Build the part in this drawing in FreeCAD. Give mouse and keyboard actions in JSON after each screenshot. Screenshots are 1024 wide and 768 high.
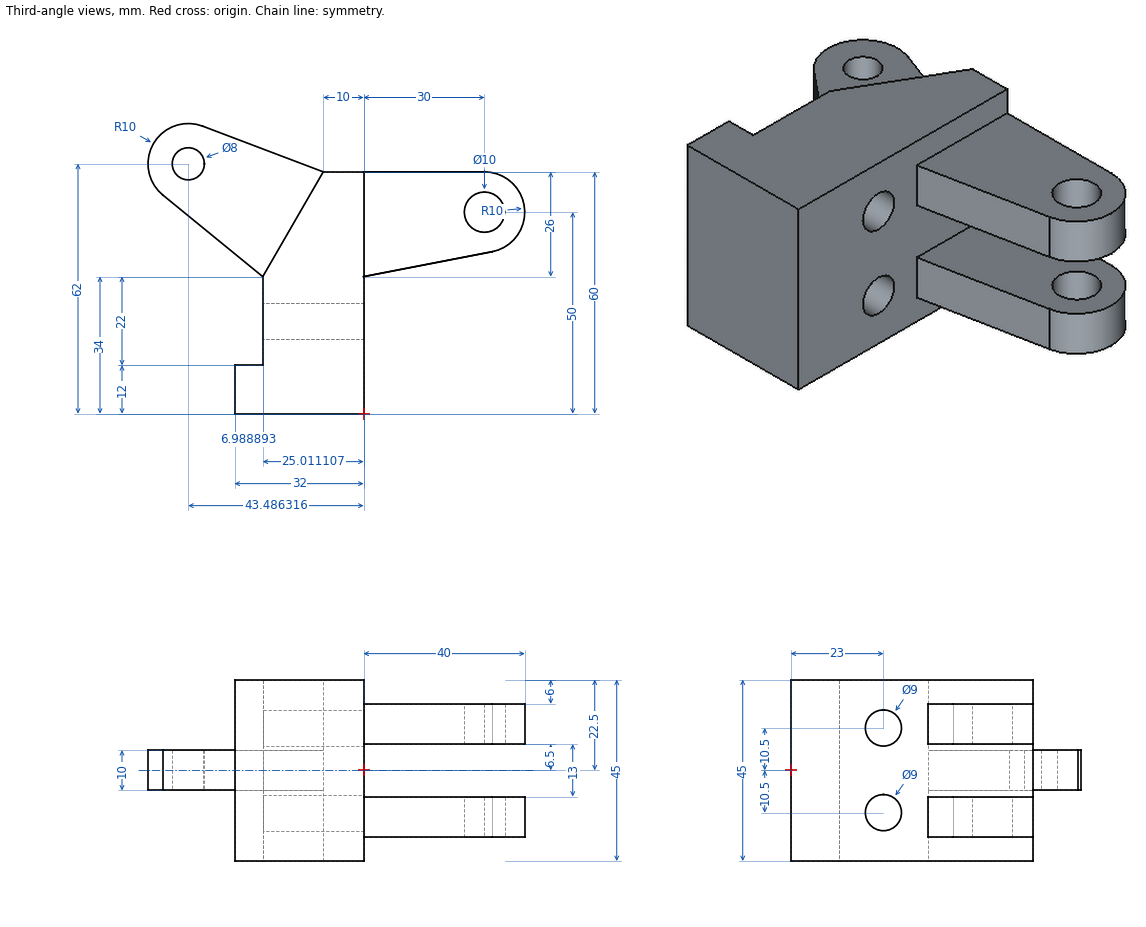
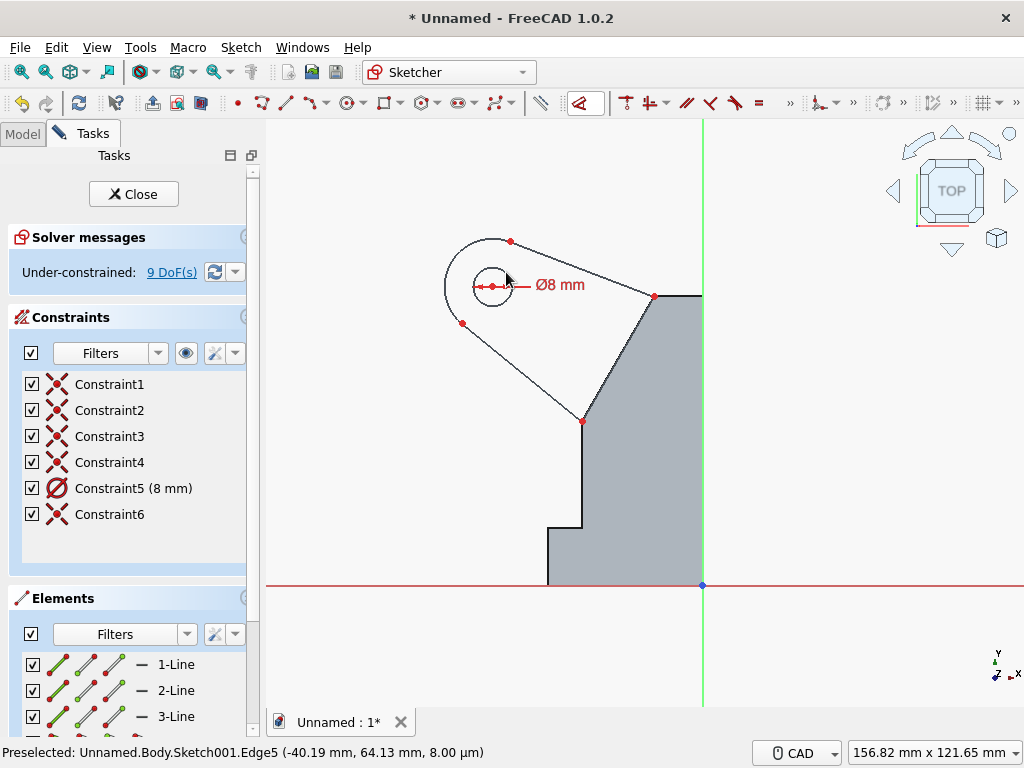
{"action": "left_click", "coordinate": [498, 353]}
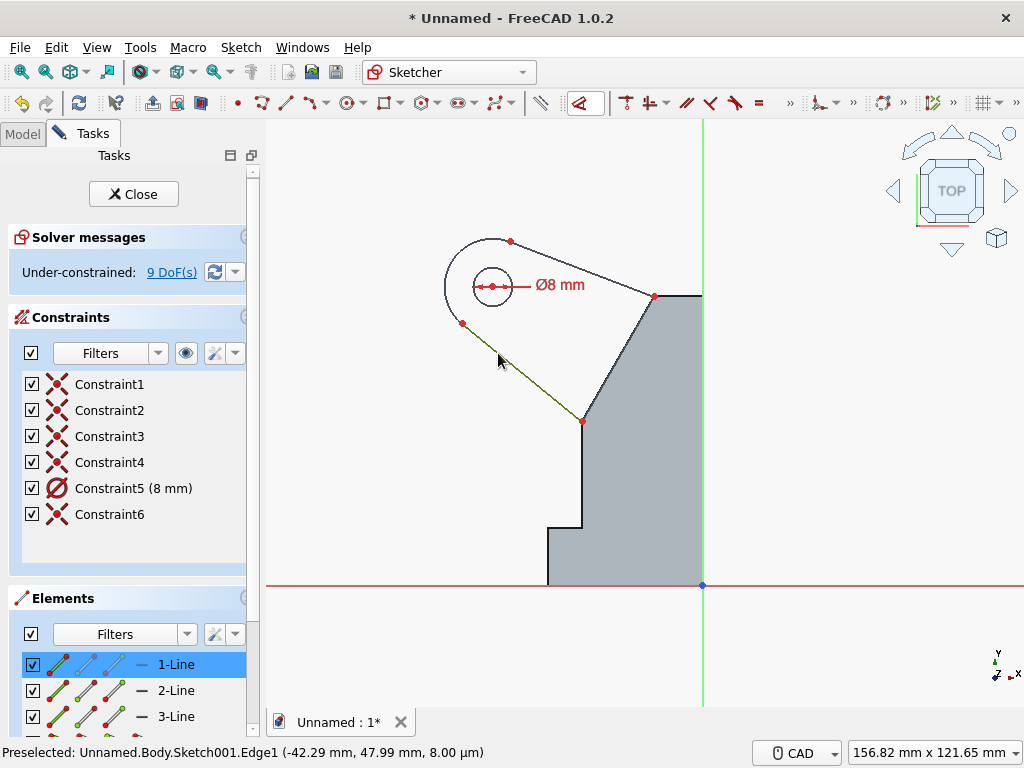
{"action": "left_click", "coordinate": [471, 244]}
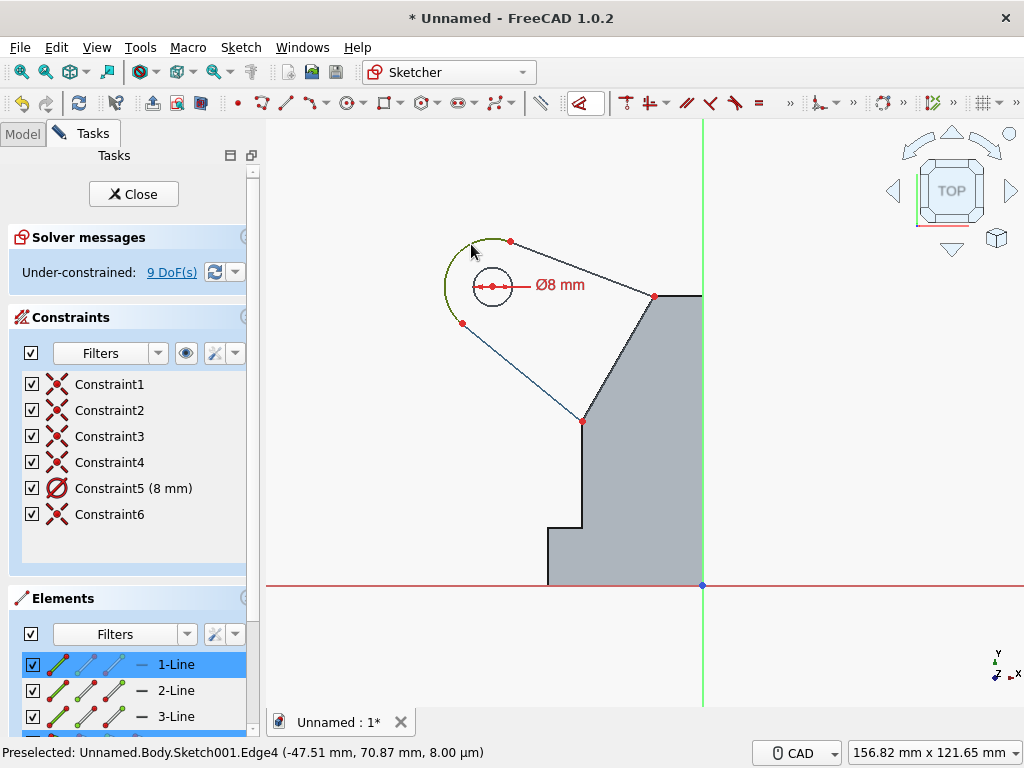
{"action": "key", "text": "t"}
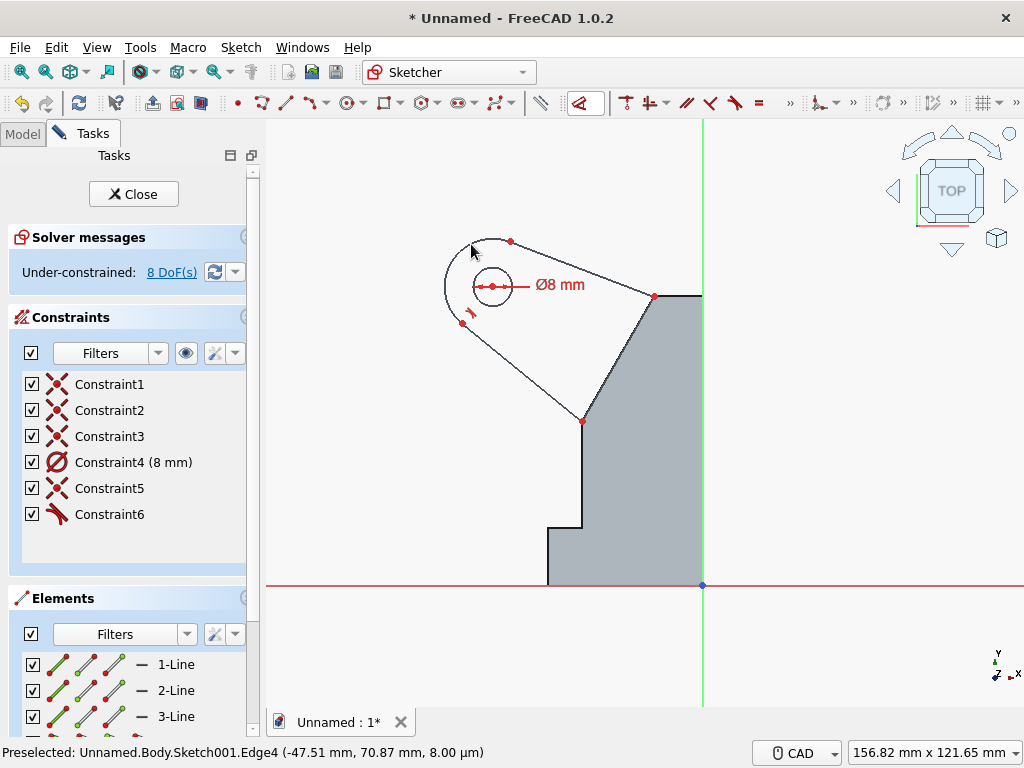
{"action": "left_click", "coordinate": [611, 281]}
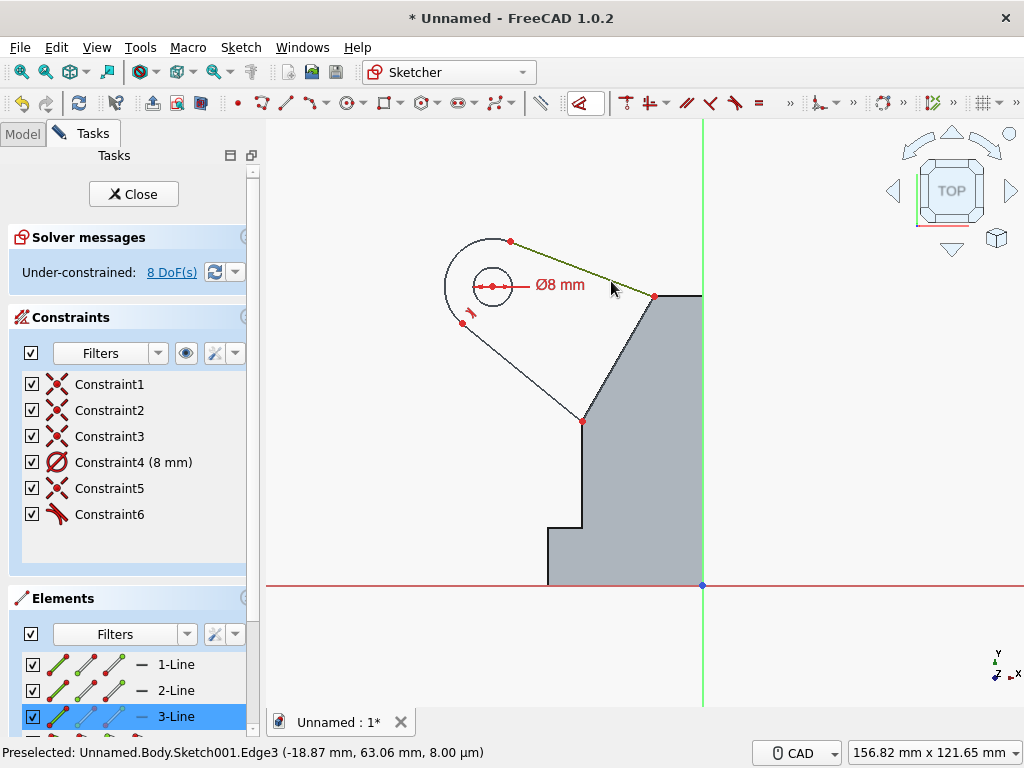
{"action": "left_click", "coordinate": [471, 244]}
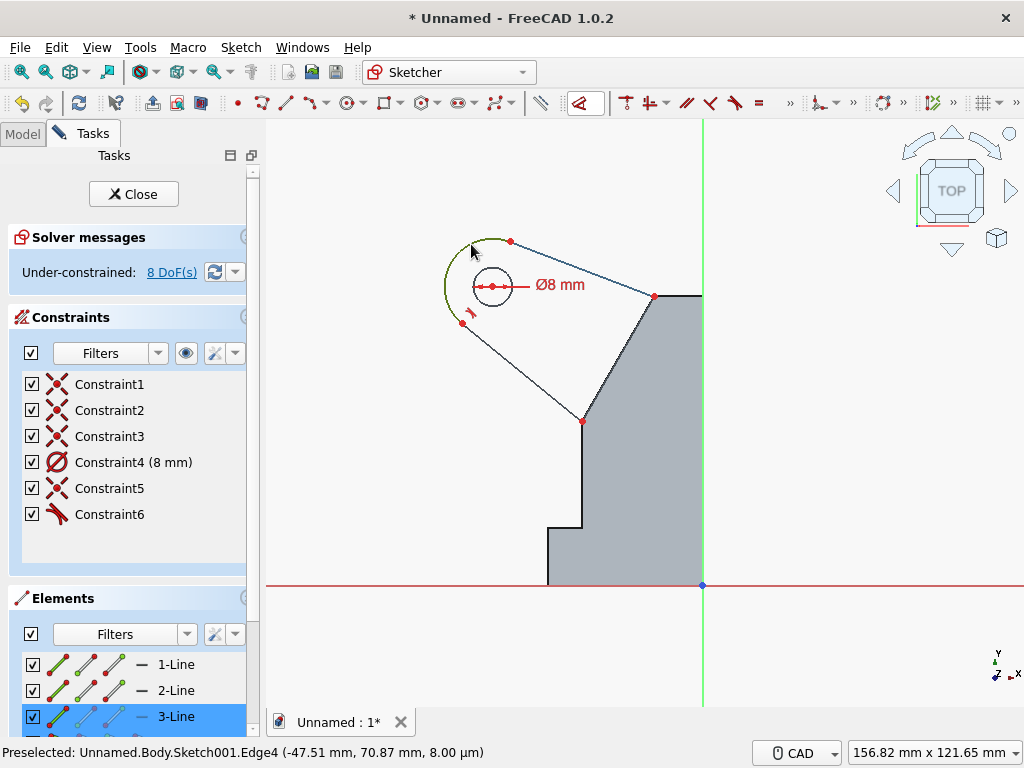
{"action": "left_click", "coordinate": [736, 104]}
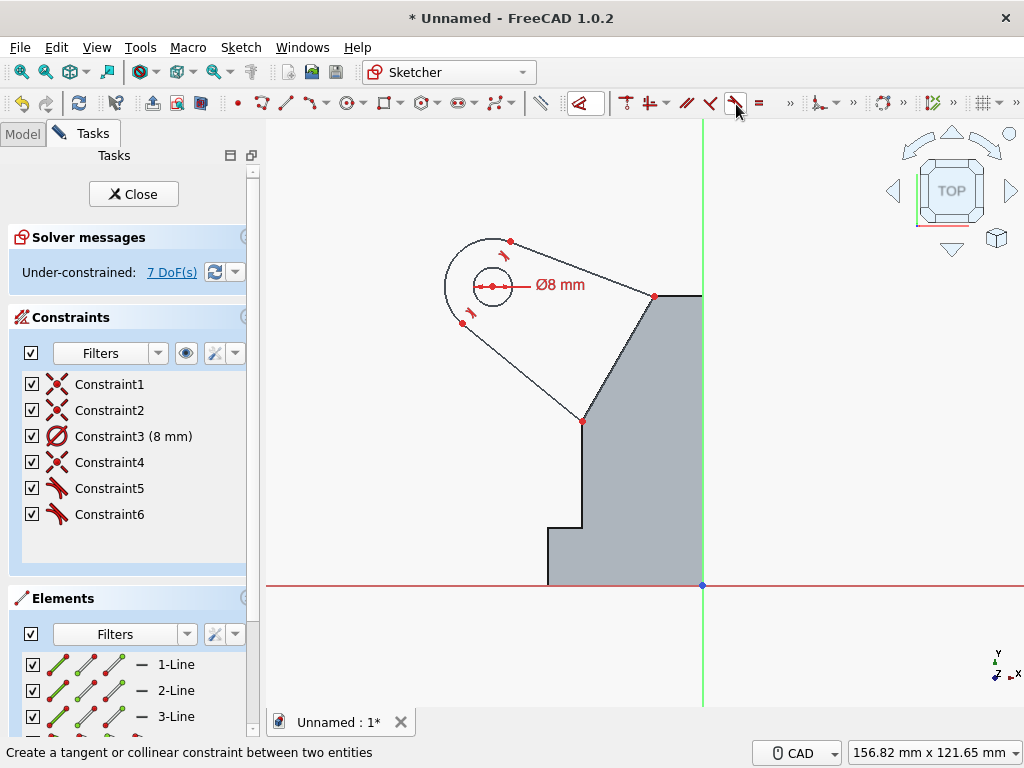
{"action": "left_click", "coordinate": [471, 244]}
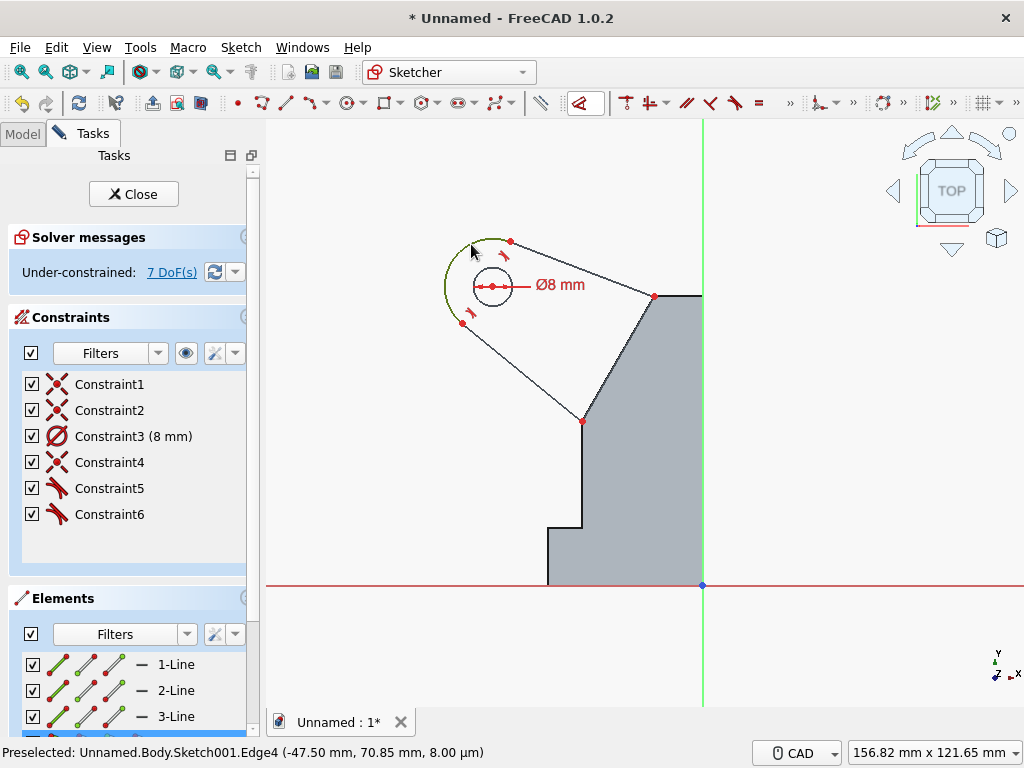
{"action": "key", "text": "k r"}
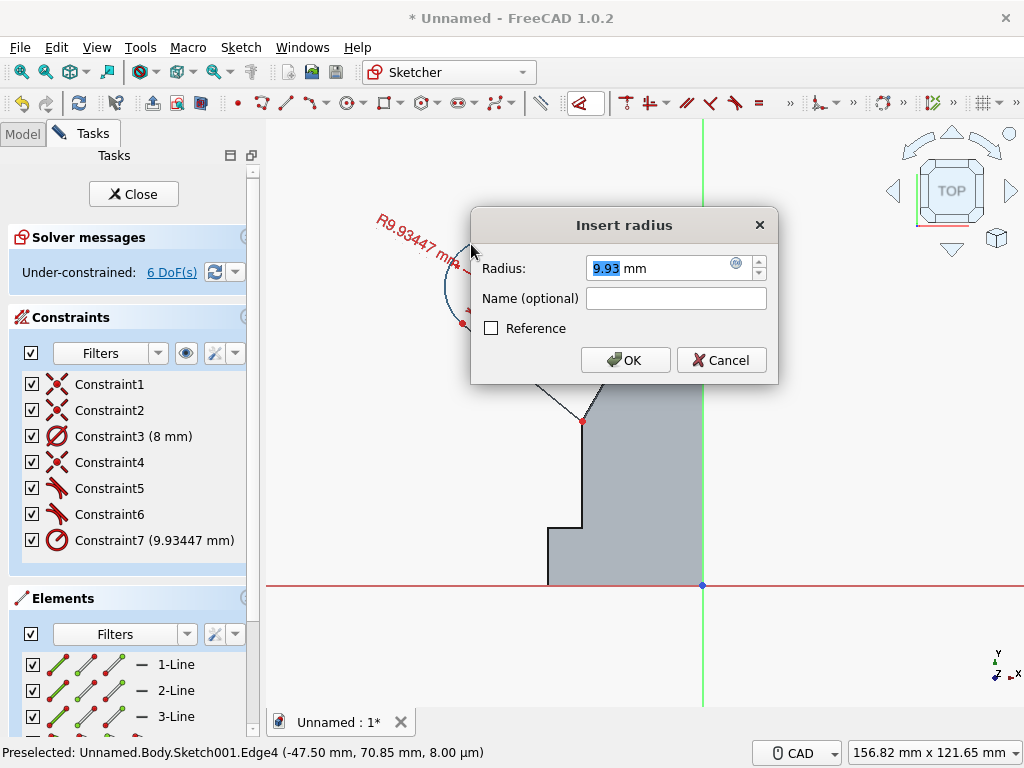
{"action": "type", "text": "10"}
{"action": "key", "text": "Return"}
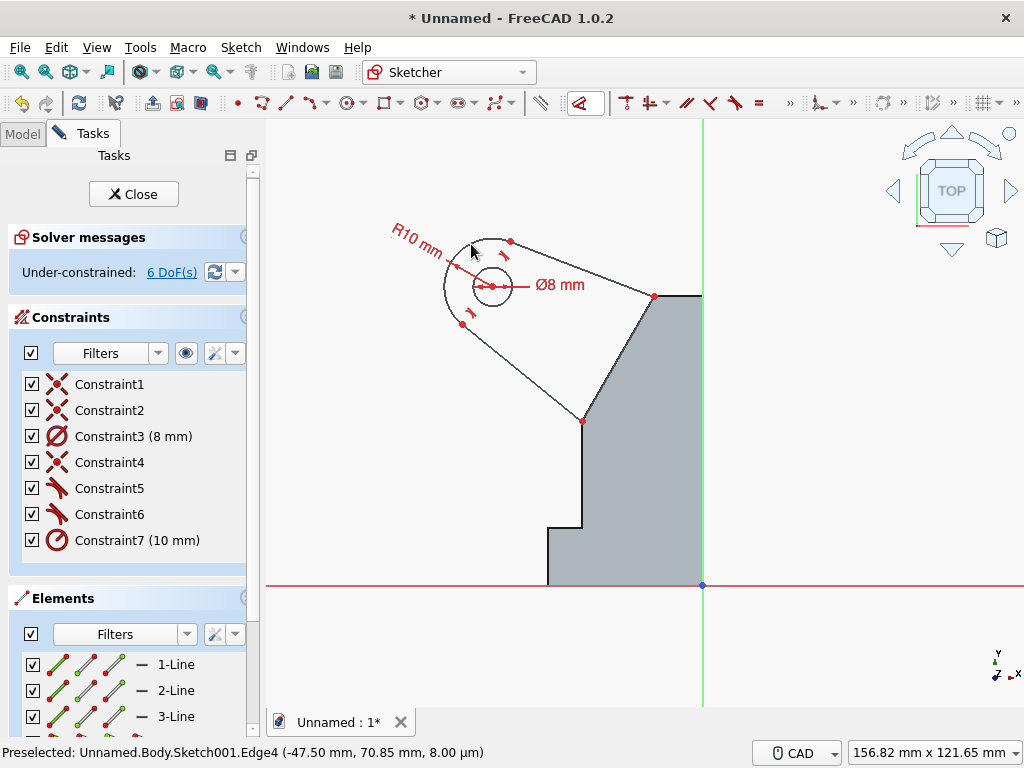
{"action": "left_click", "coordinate": [493, 287]}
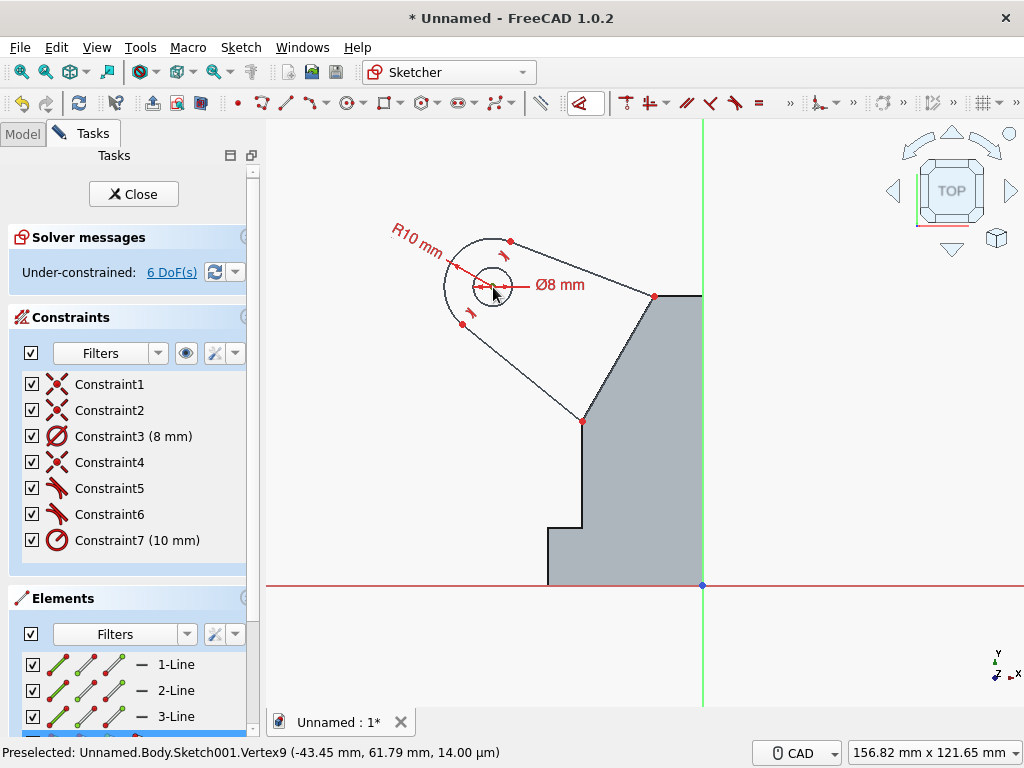
{"action": "key", "text": "i"}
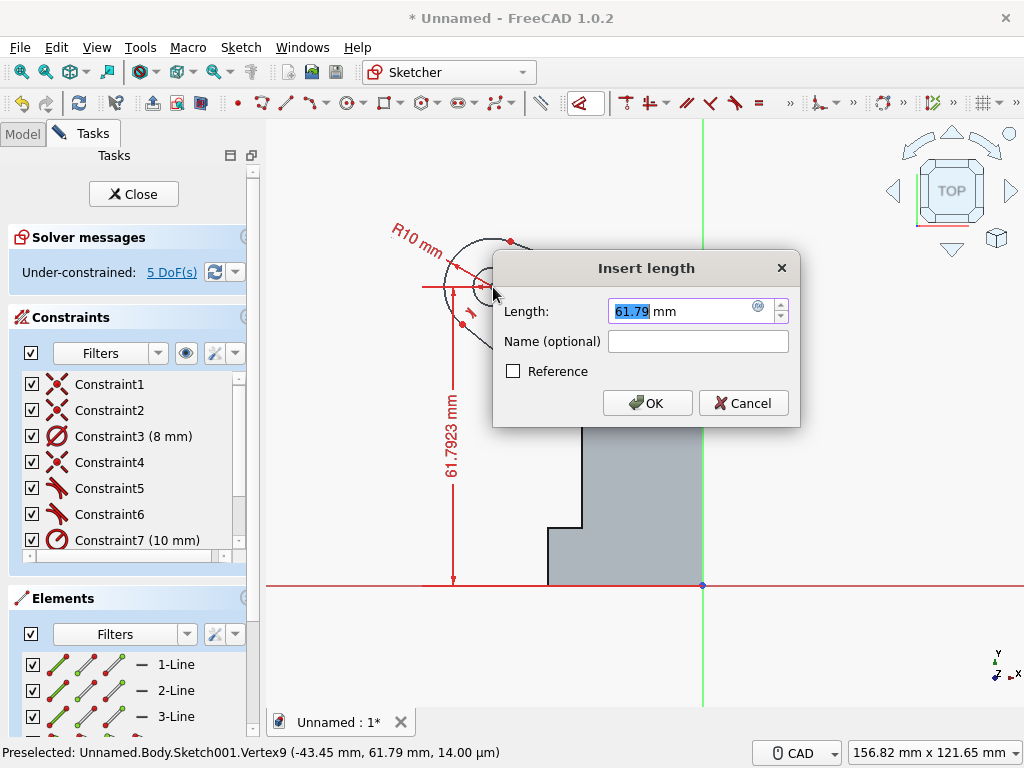
{"action": "type", "text": "62"}
{"action": "key", "text": "Return"}